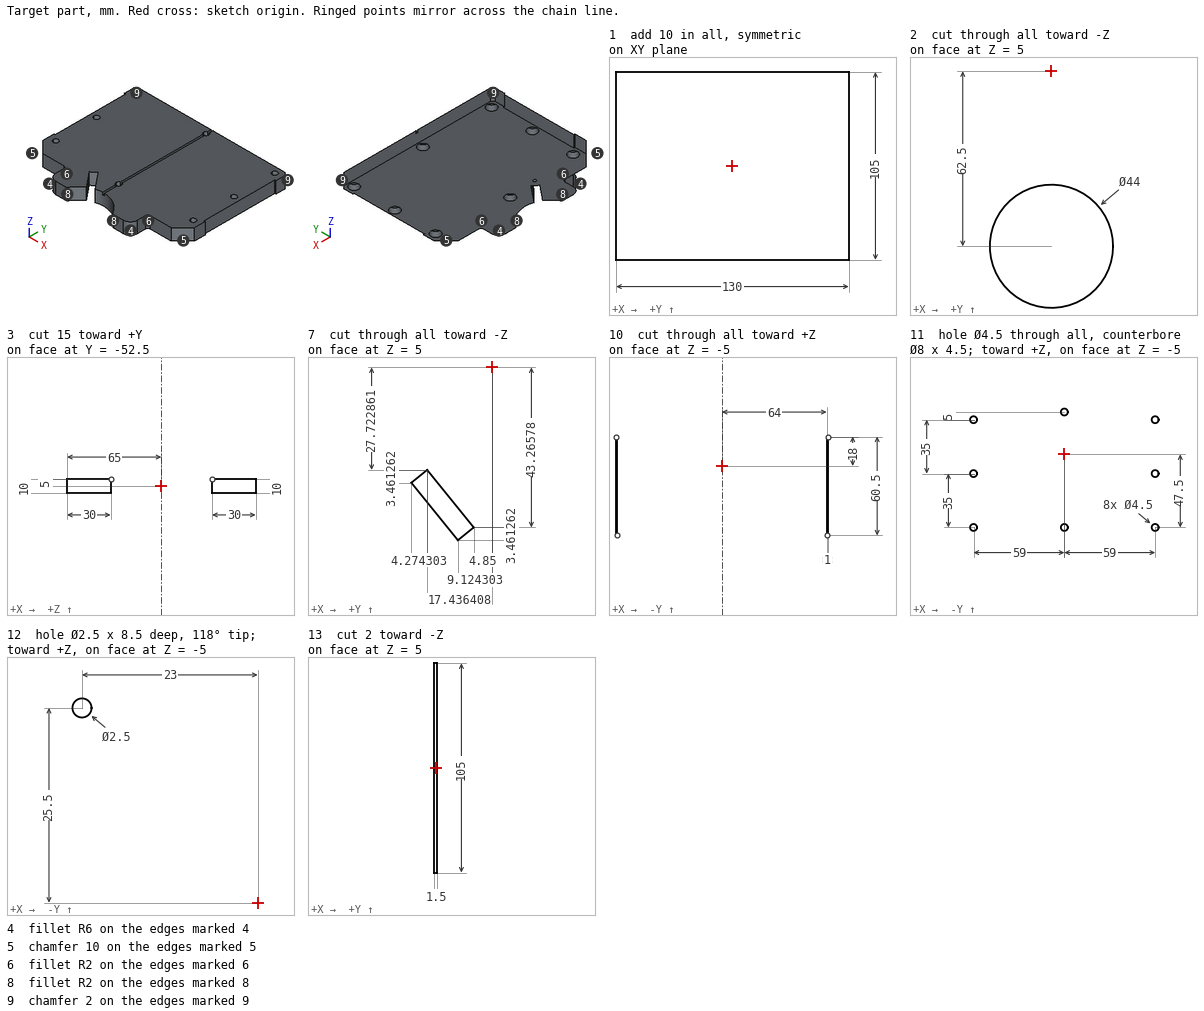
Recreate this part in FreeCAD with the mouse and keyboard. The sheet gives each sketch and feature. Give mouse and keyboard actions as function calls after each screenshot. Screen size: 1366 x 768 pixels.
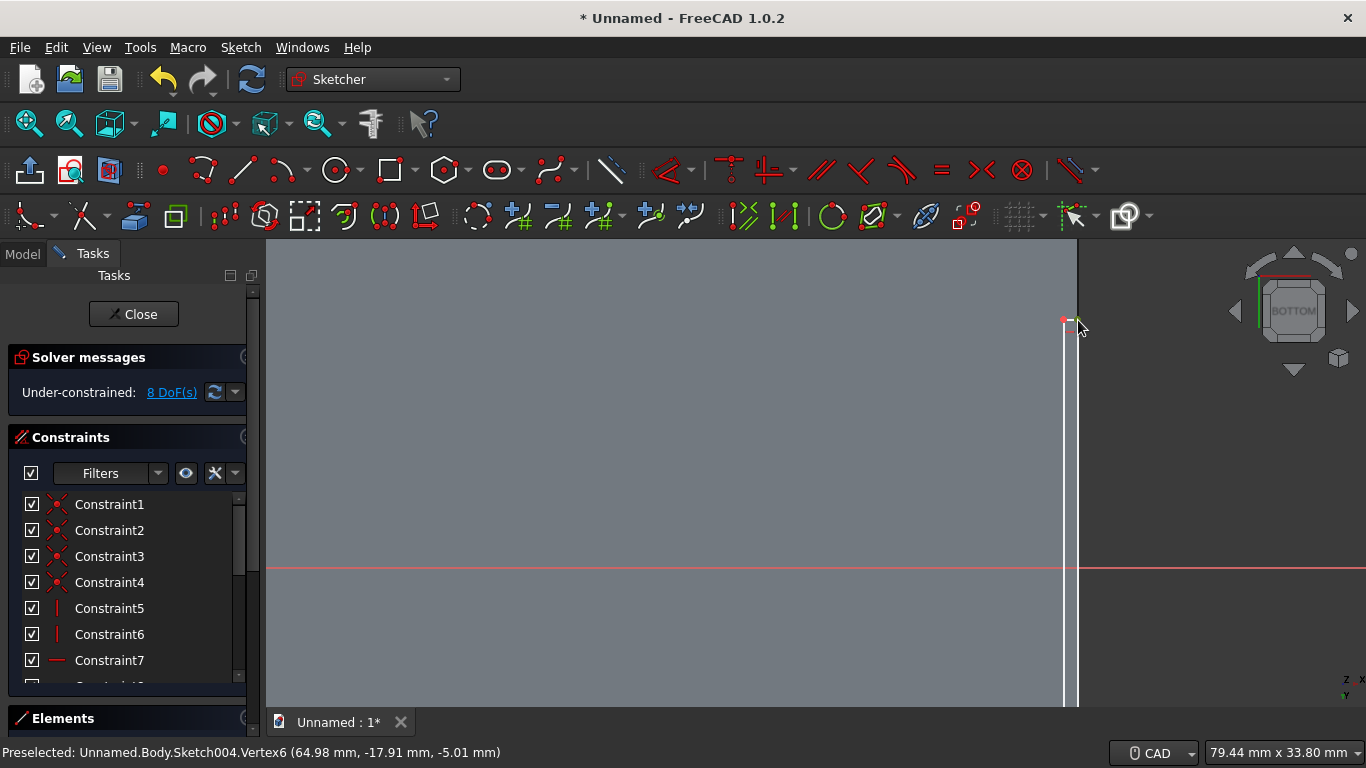
scroll(1079, 319, down, 5)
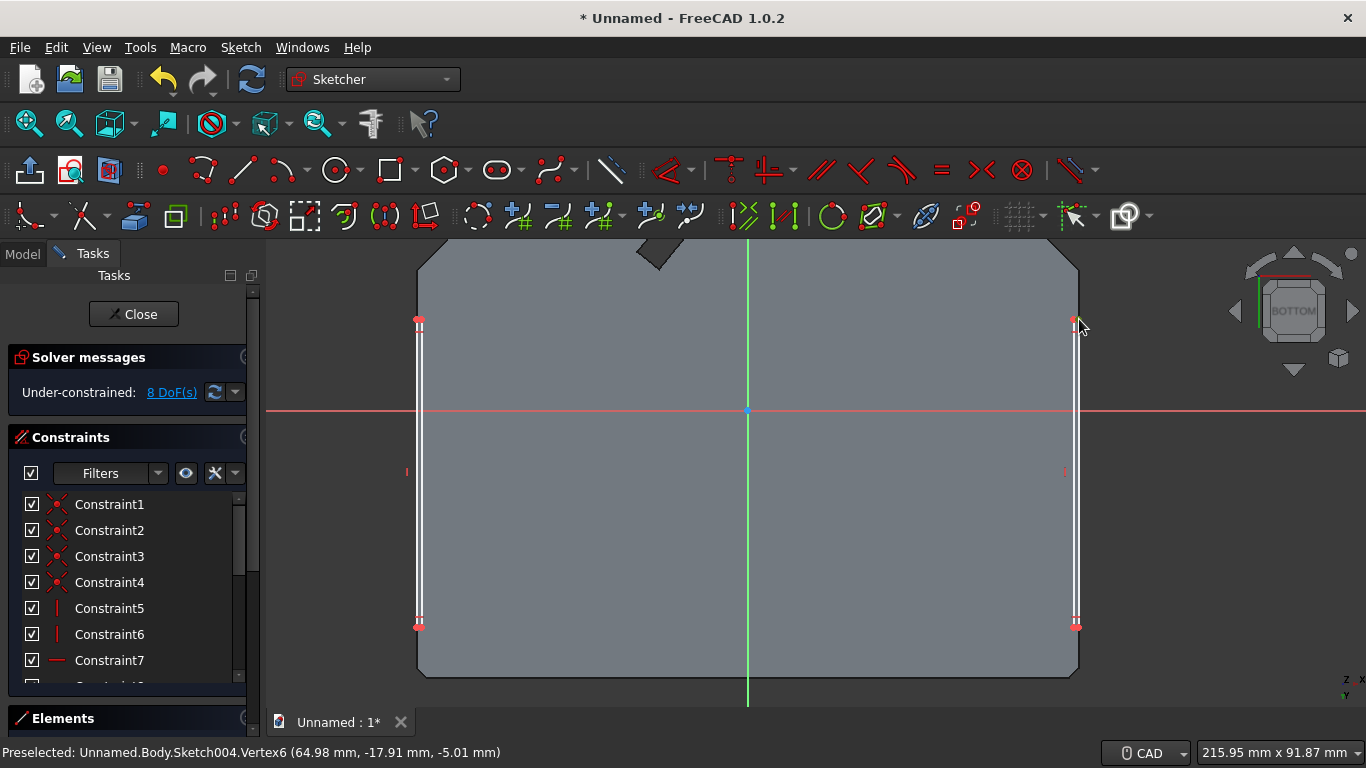
scroll(417, 319, up, 5)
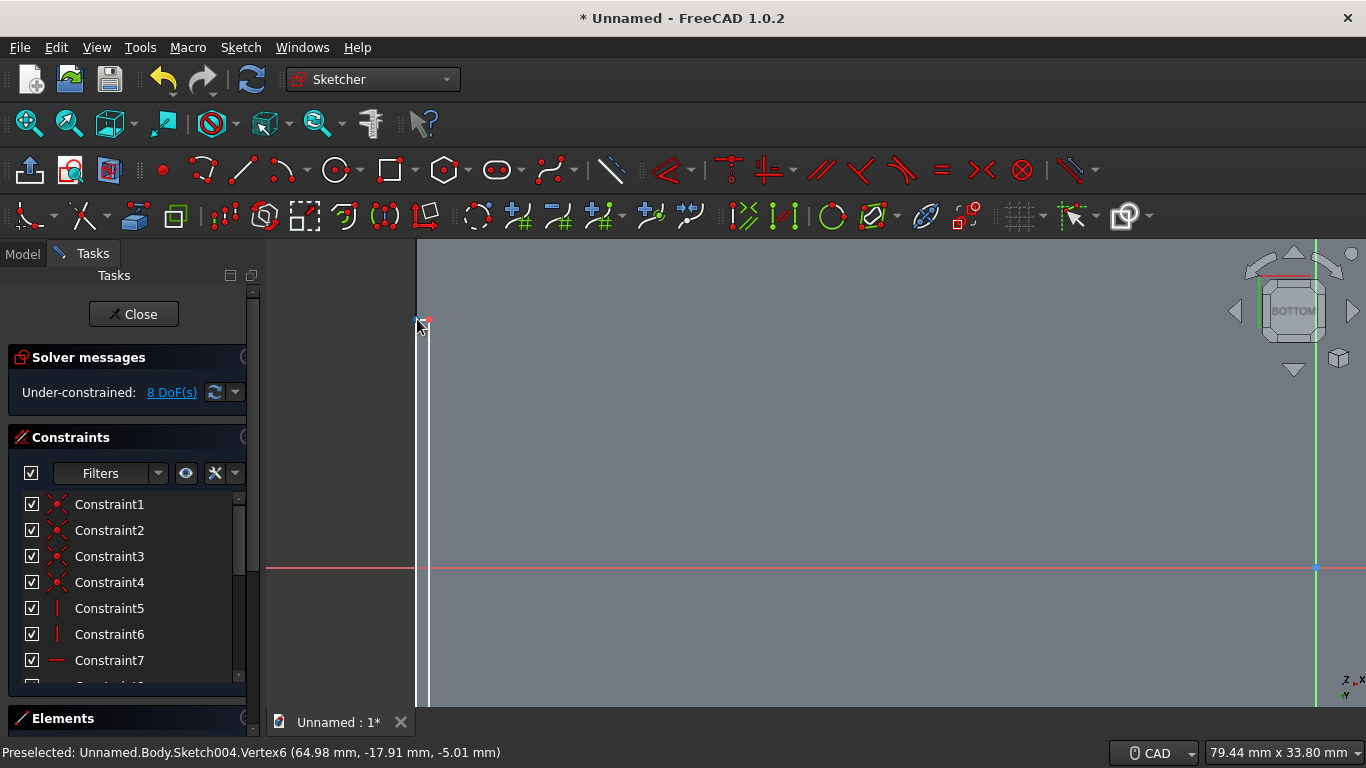
click(416, 320)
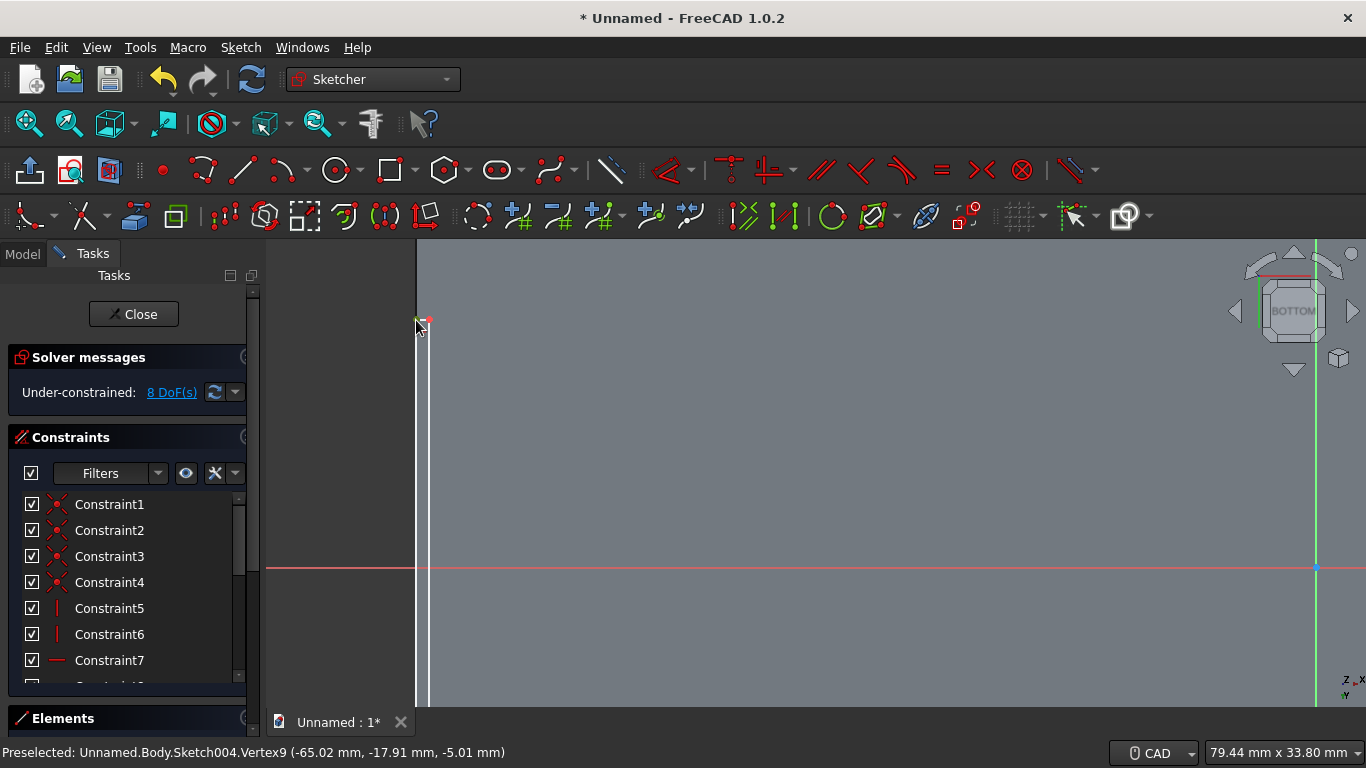
scroll(416, 319, down, 5)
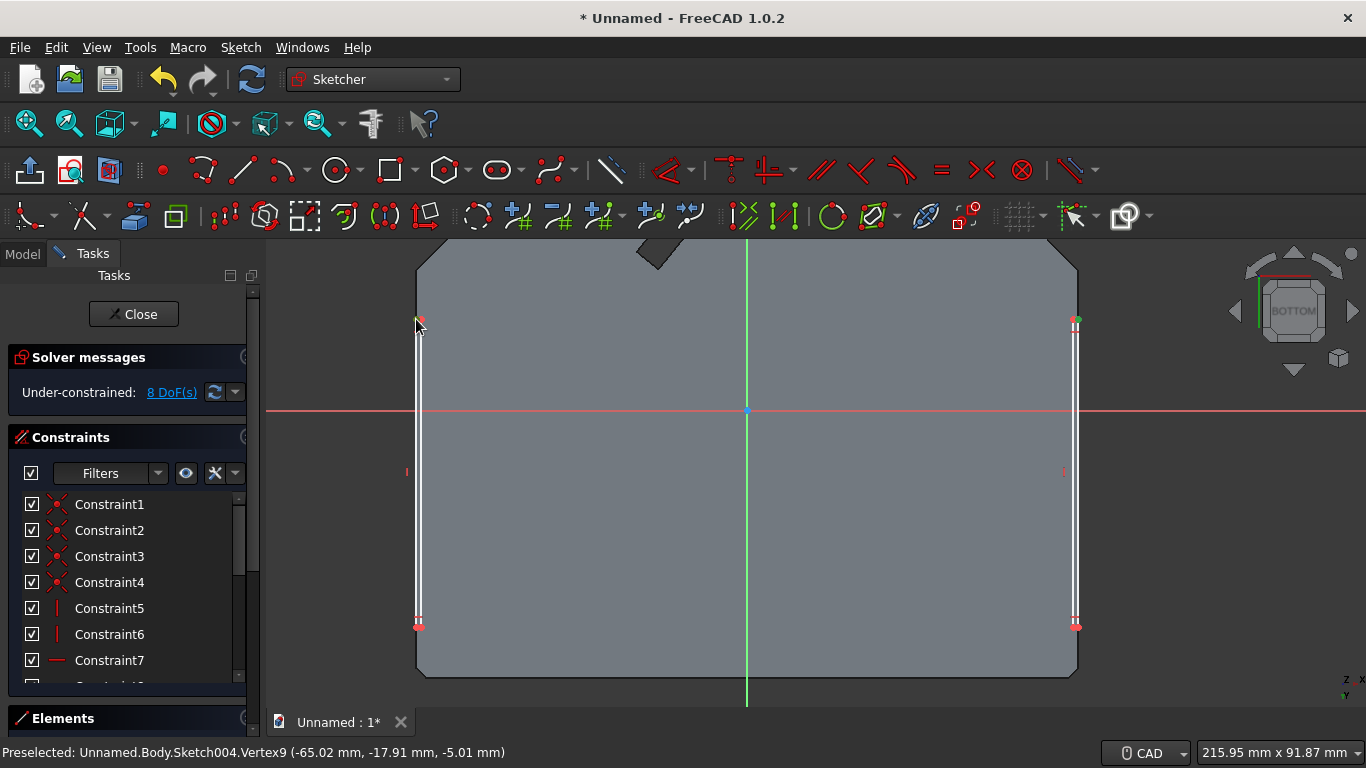
click(747, 650)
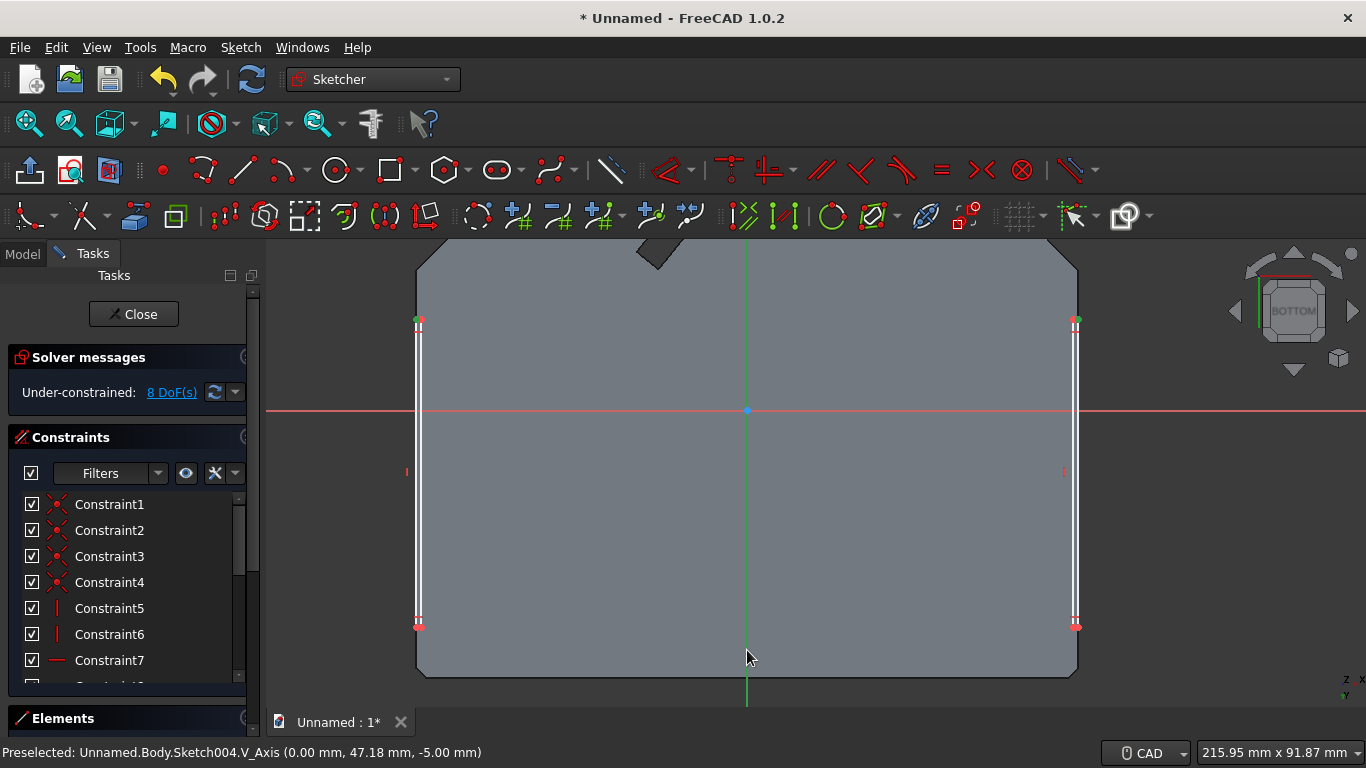
click(982, 170)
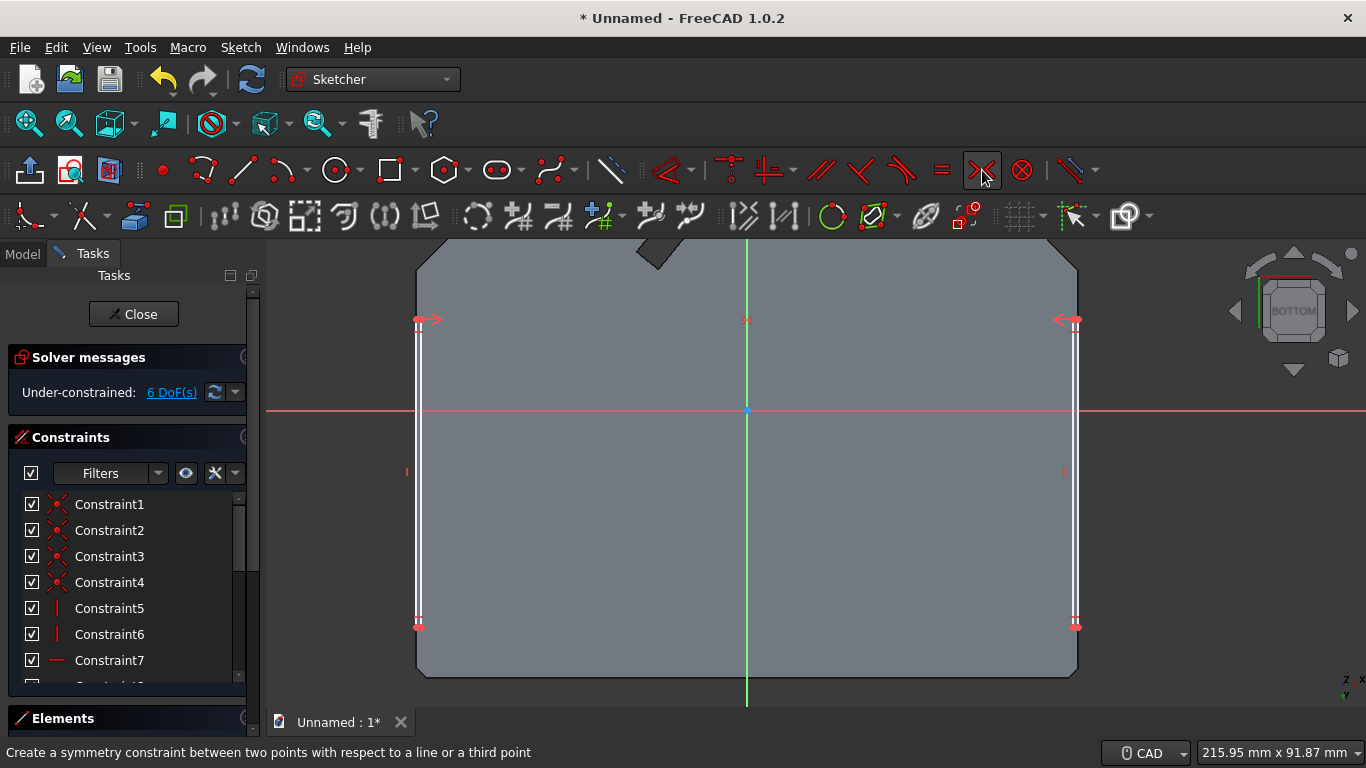
scroll(1073, 628, up, 5)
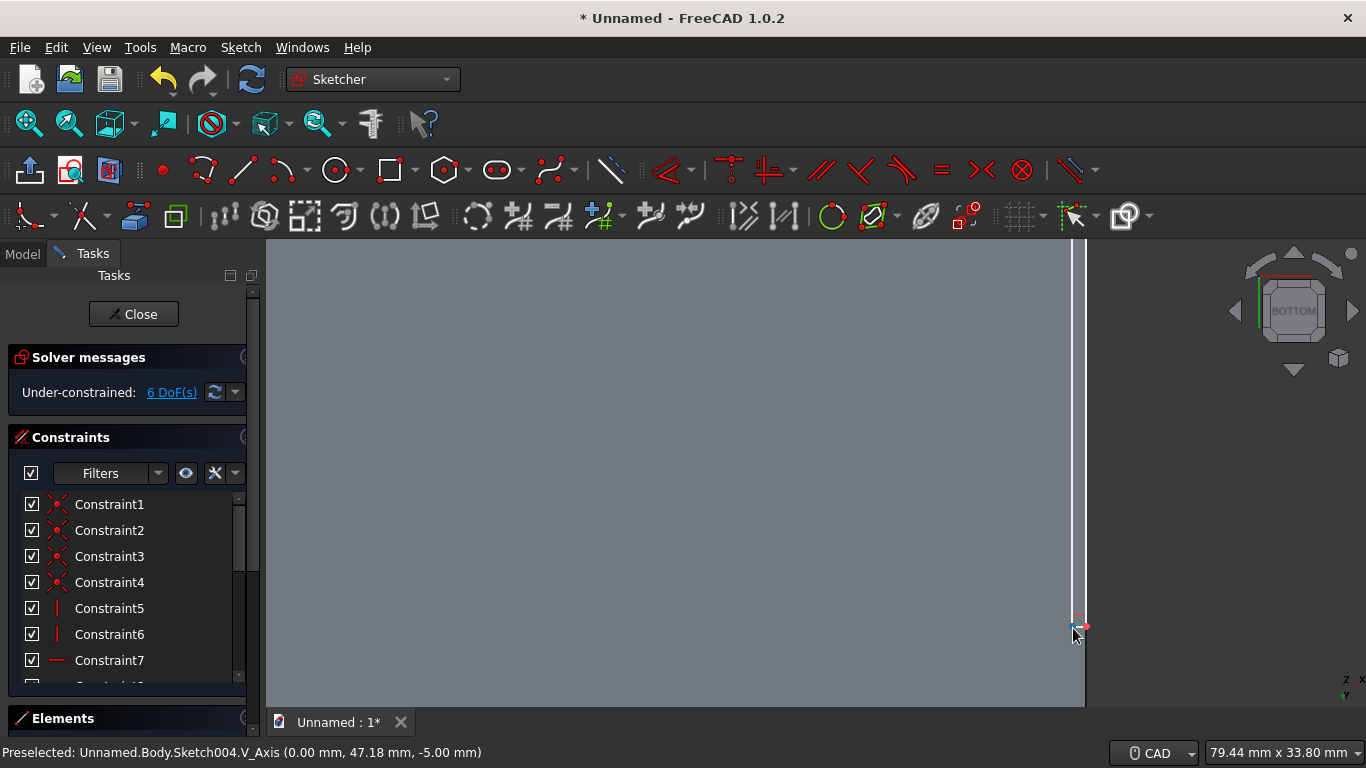
click(1072, 627)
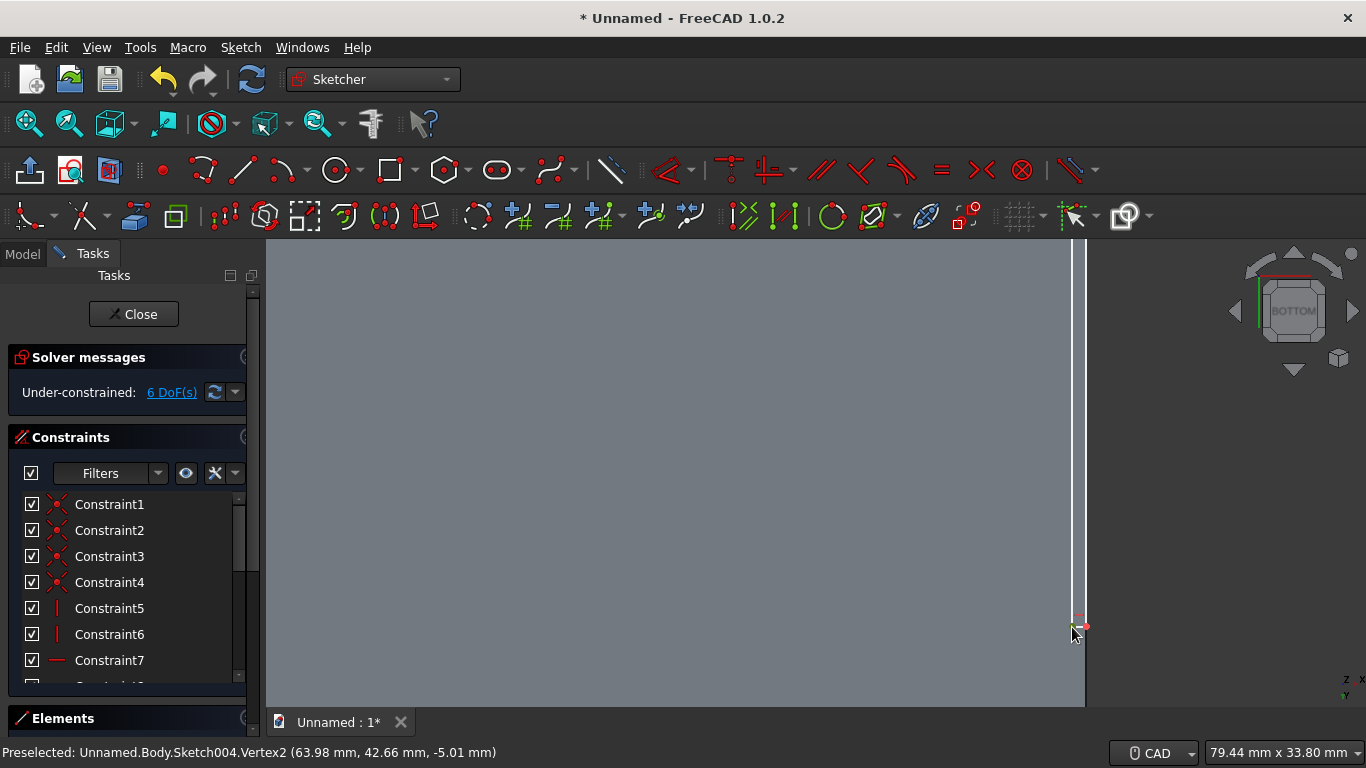
scroll(1074, 629, down, 5)